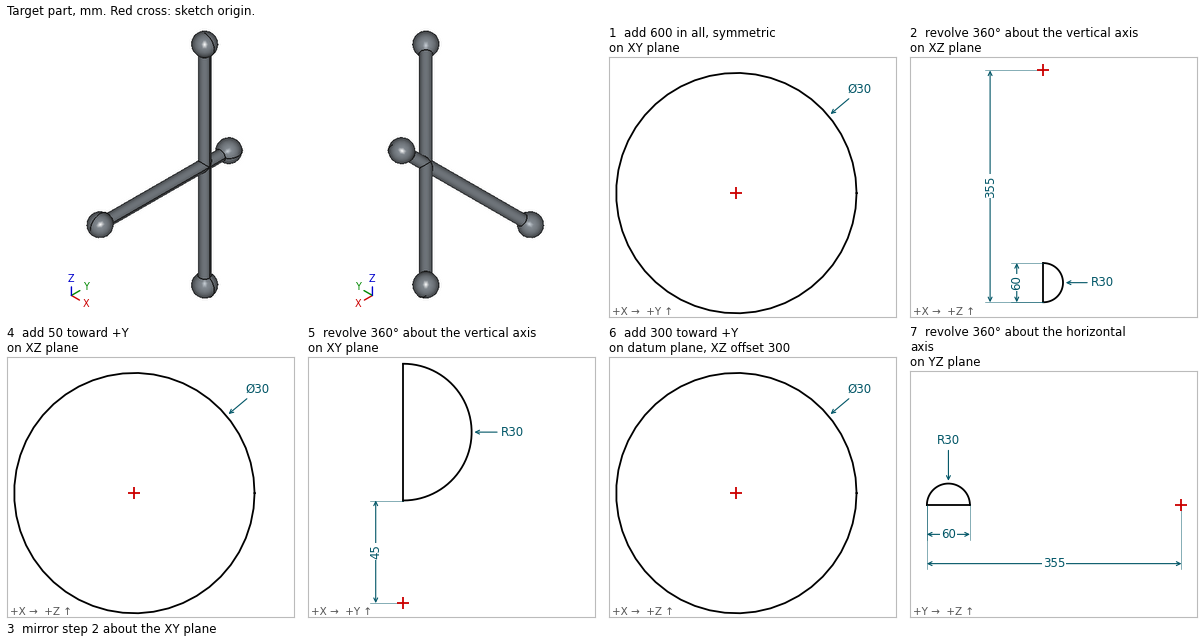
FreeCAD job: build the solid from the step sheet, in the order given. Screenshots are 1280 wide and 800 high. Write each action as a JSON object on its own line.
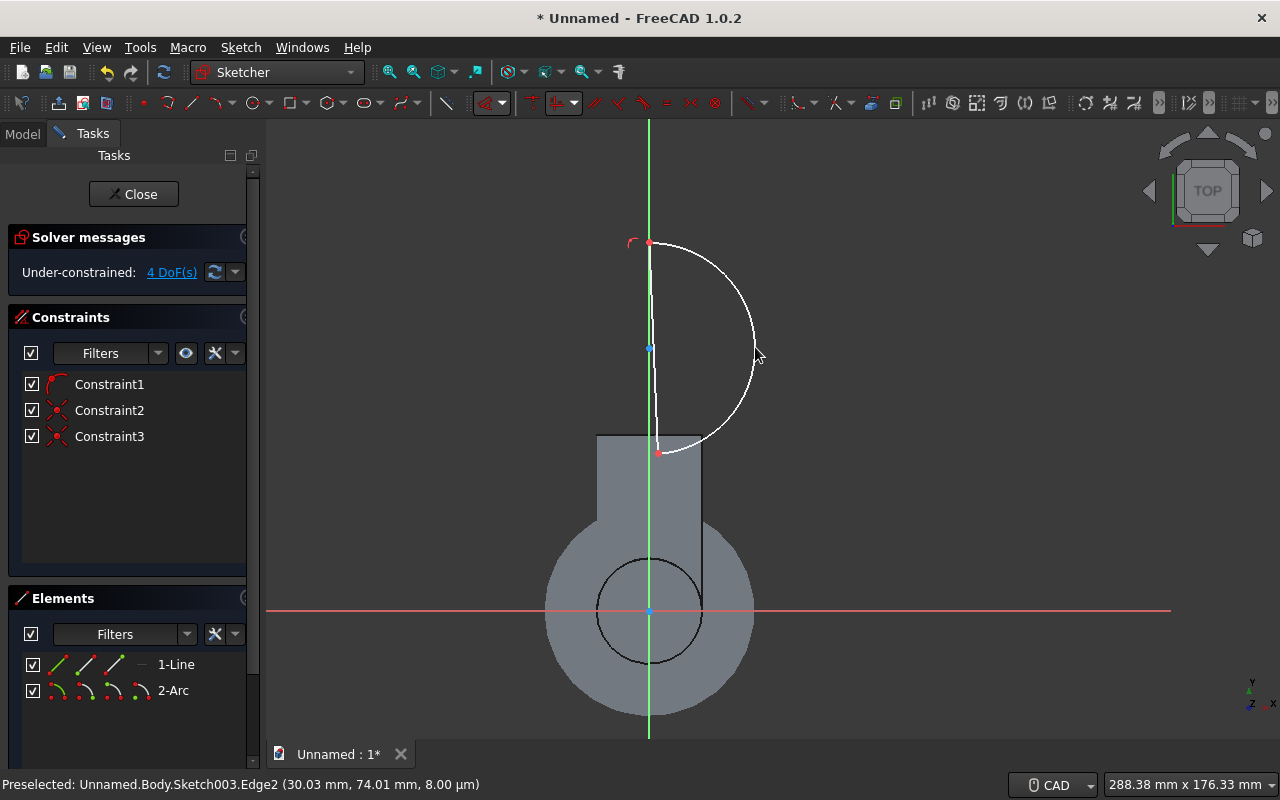
{"action": "left_click", "coordinate": [652, 306]}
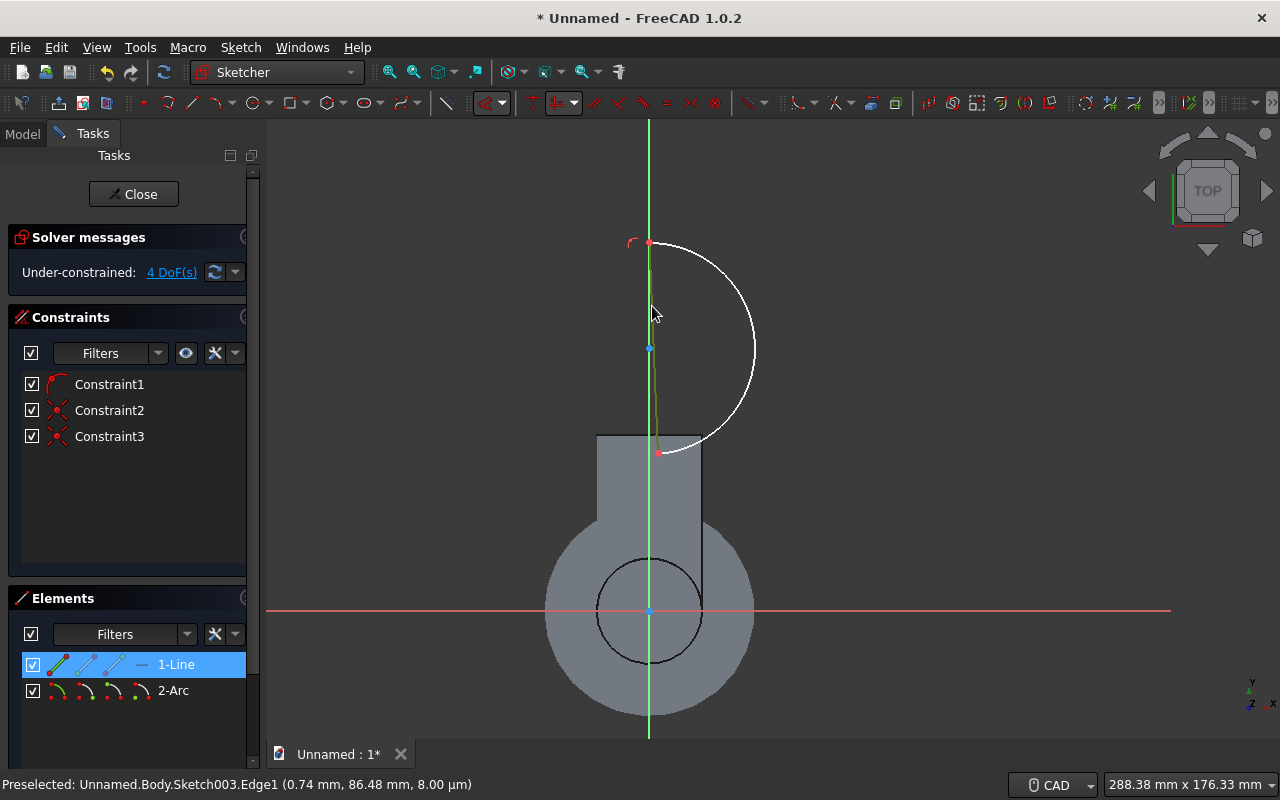
{"action": "left_click", "coordinate": [576, 104]}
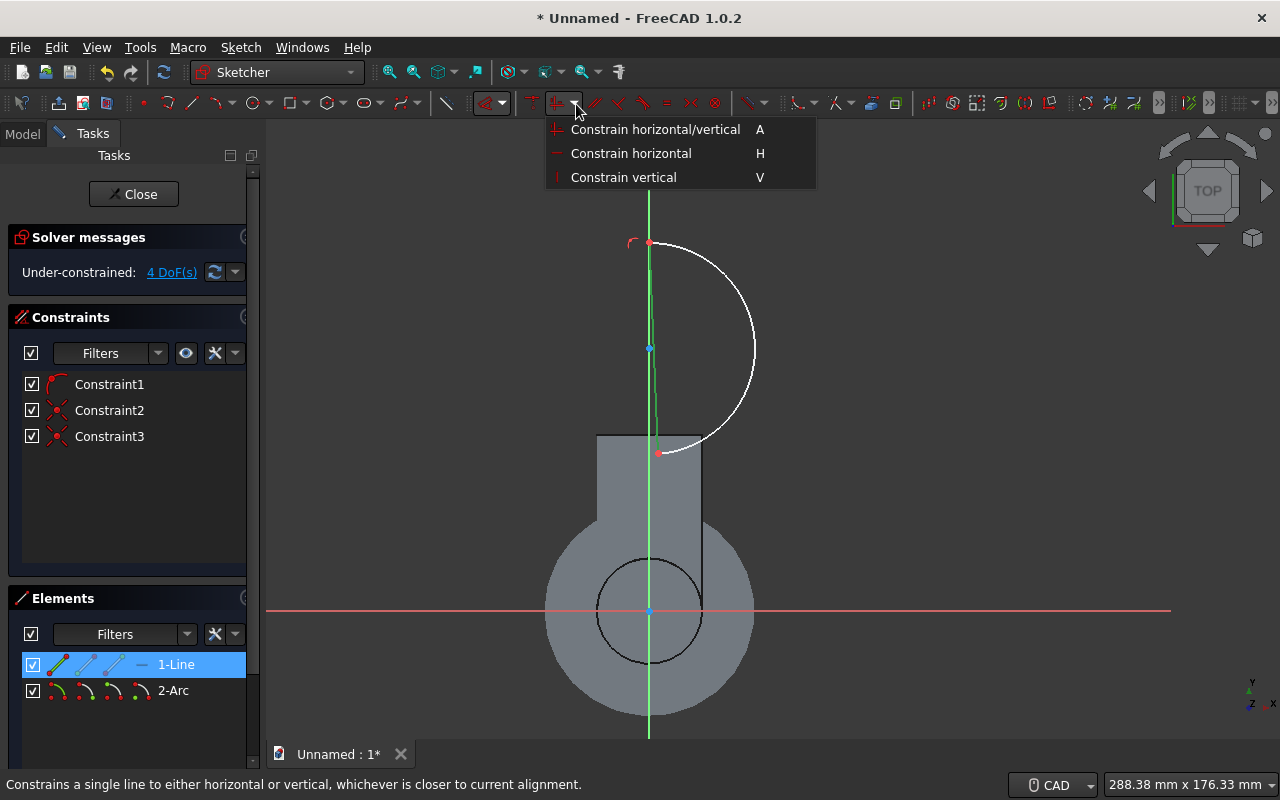
{"action": "left_click", "coordinate": [681, 177]}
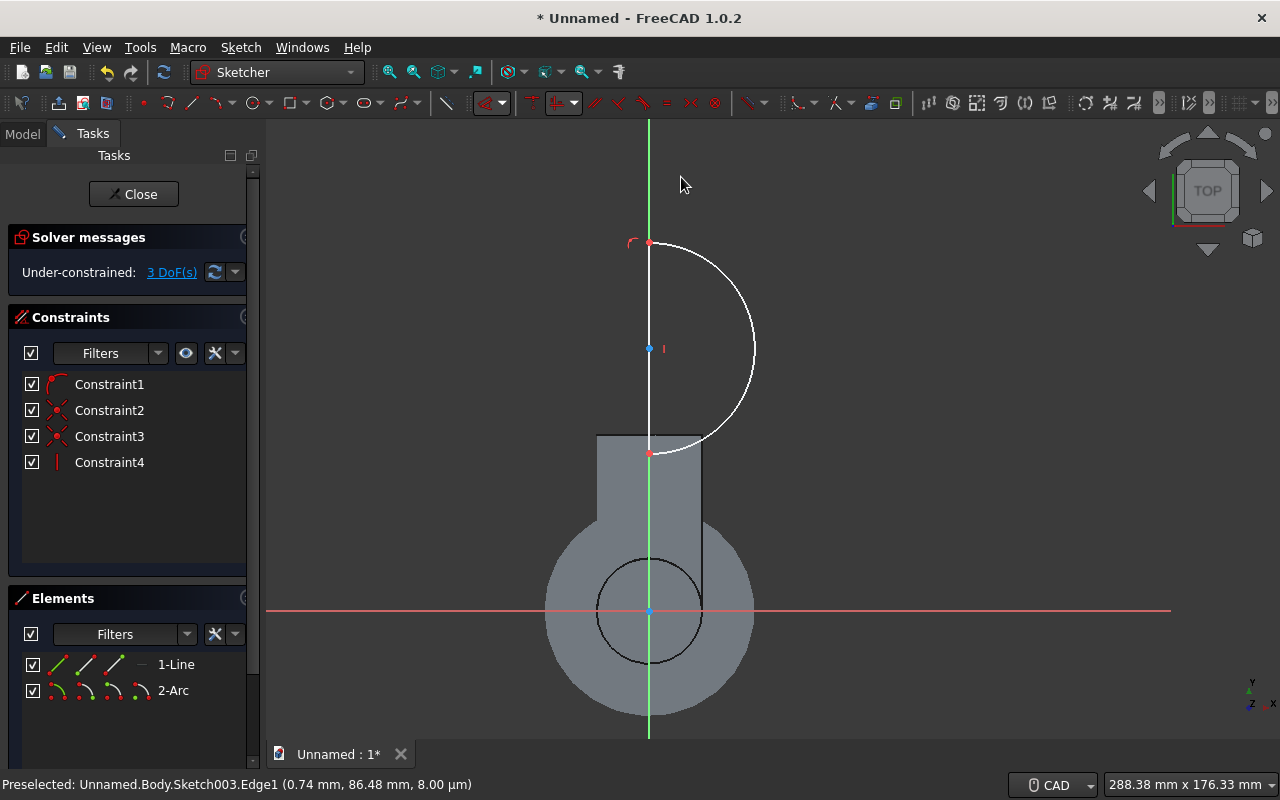
{"action": "left_click", "coordinate": [649, 348]}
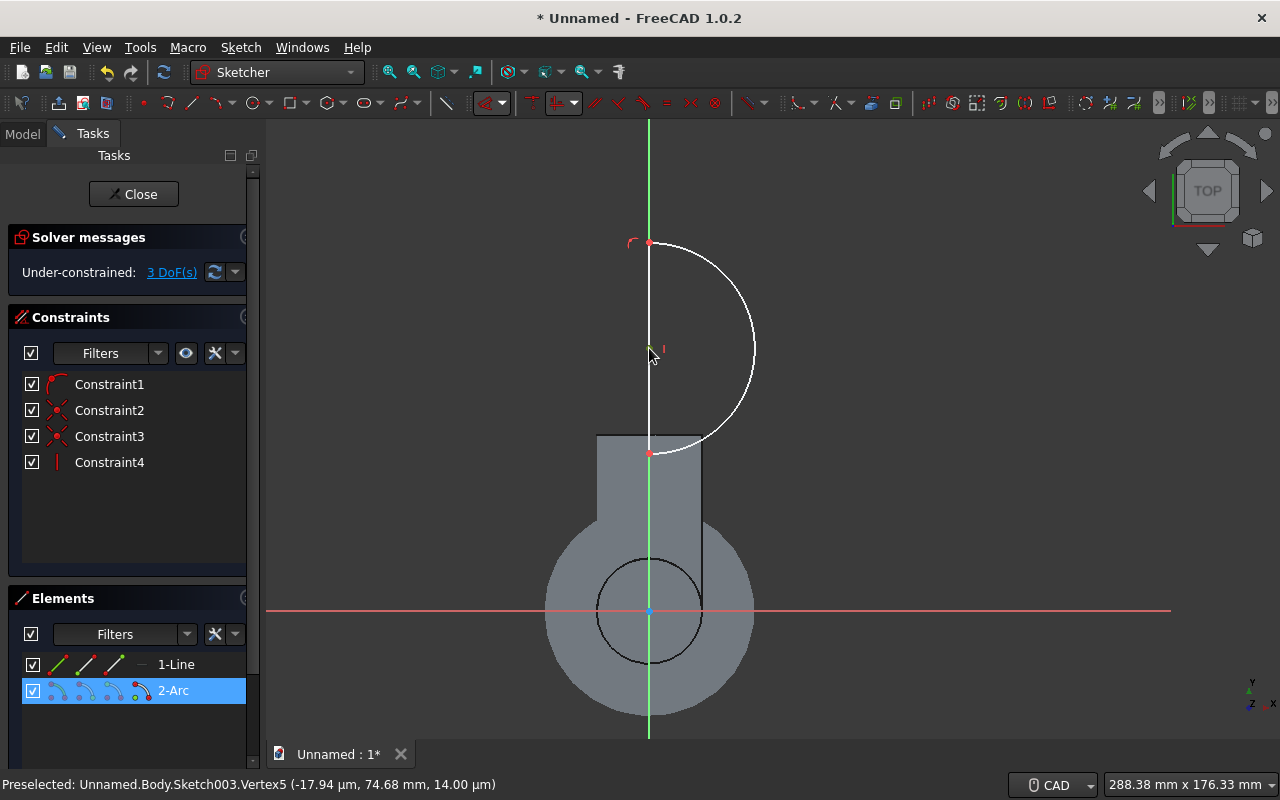
{"action": "left_click", "coordinate": [649, 671]}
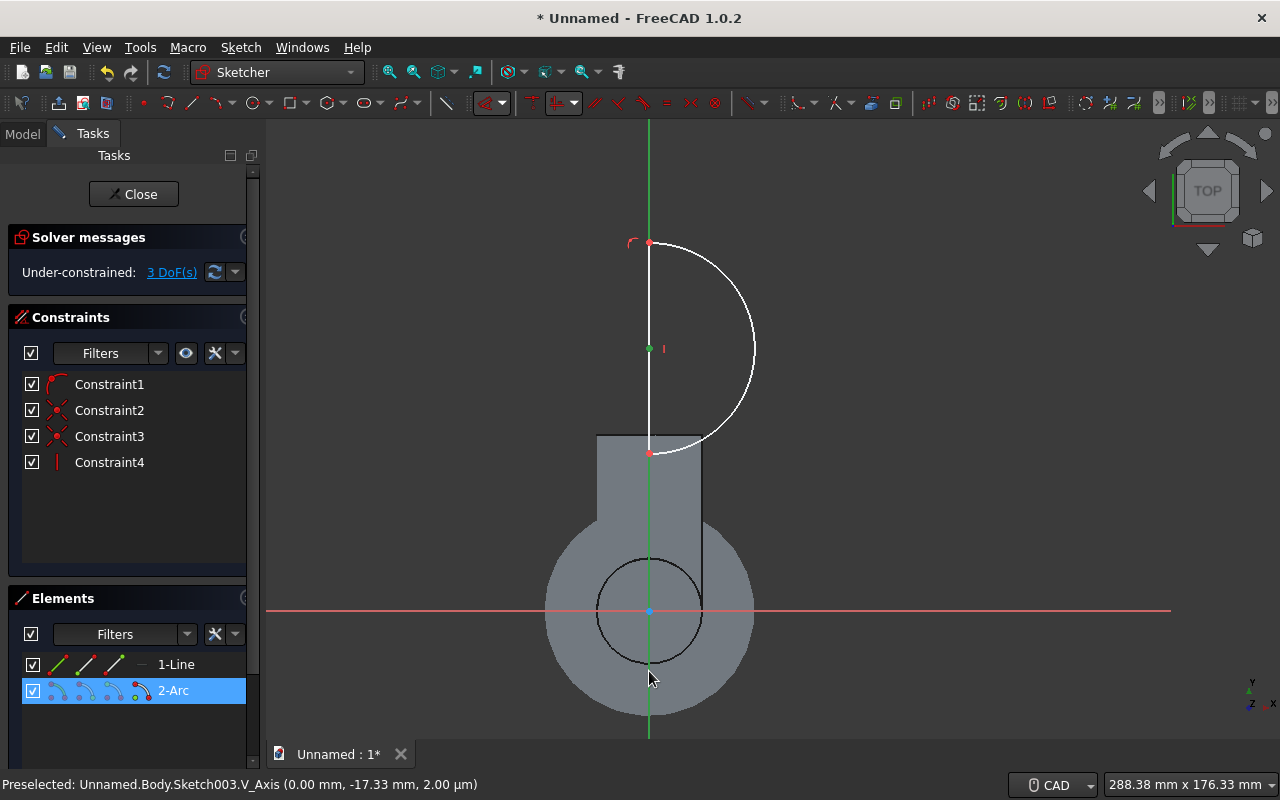
{"action": "left_click", "coordinate": [532, 104]}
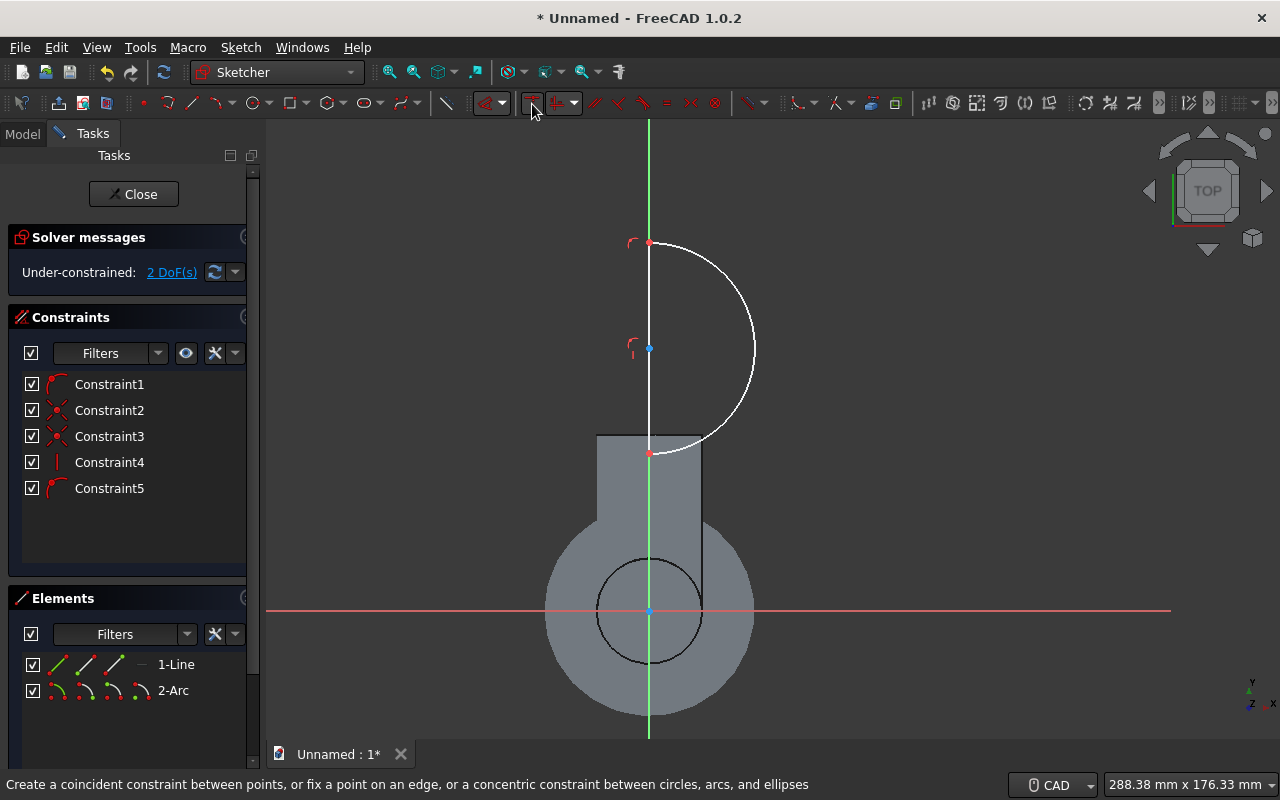
{"action": "left_click", "coordinate": [735, 411]}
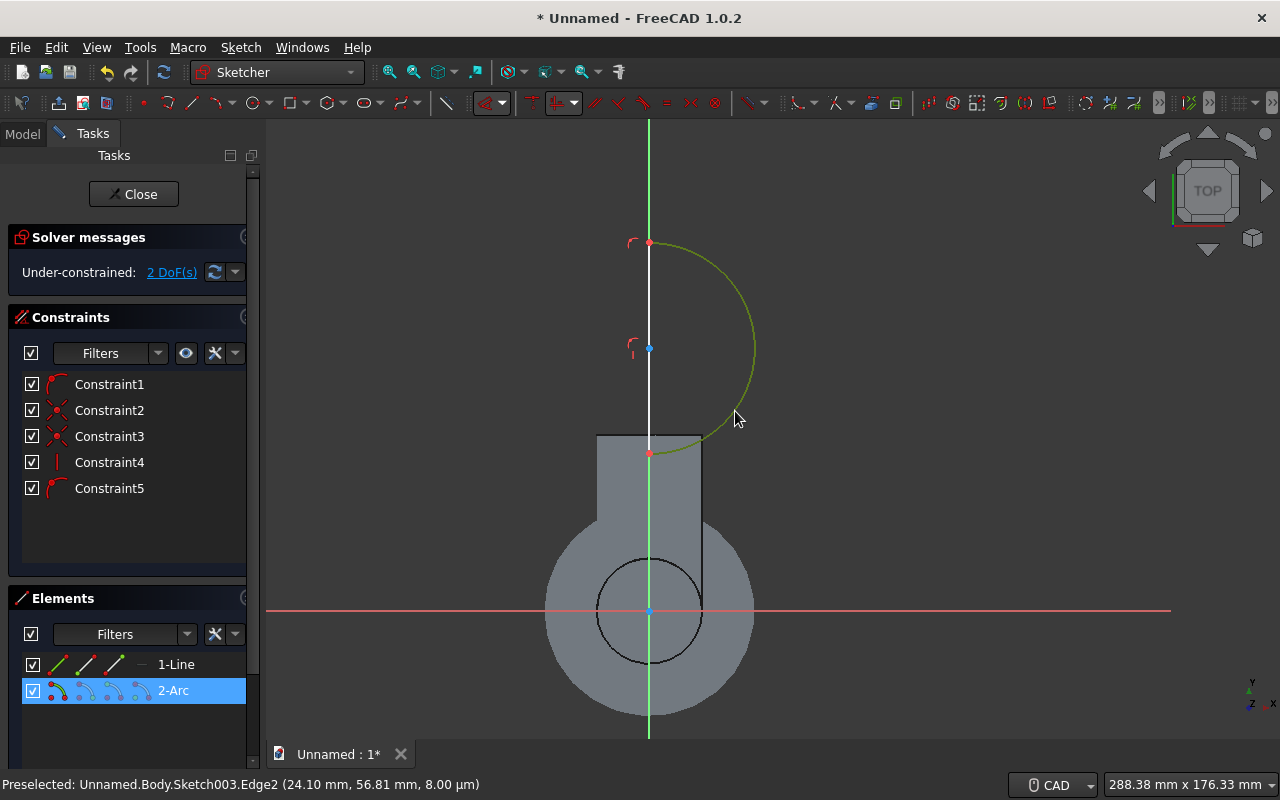
{"action": "left_click", "coordinate": [504, 104]}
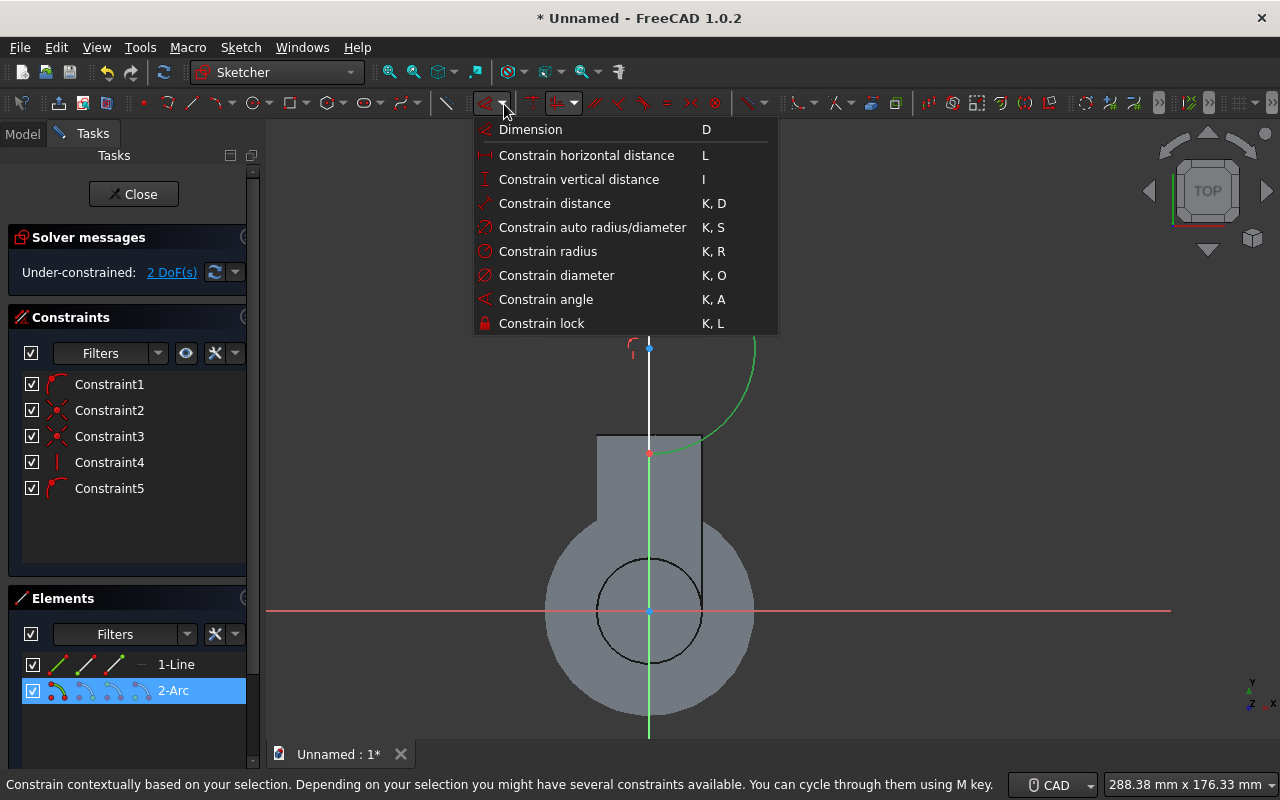
{"action": "left_click", "coordinate": [626, 251]}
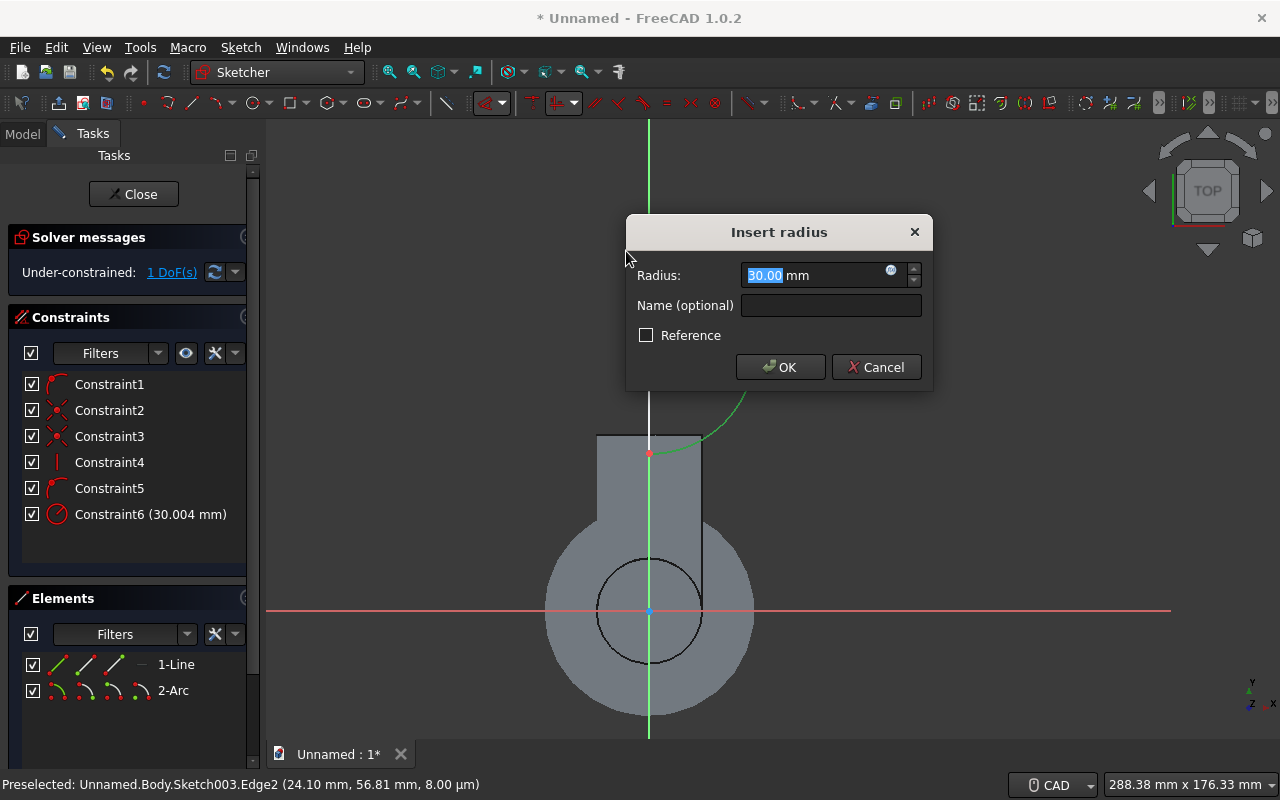
{"action": "type", "text": "30"}
{"action": "key", "text": "Return"}